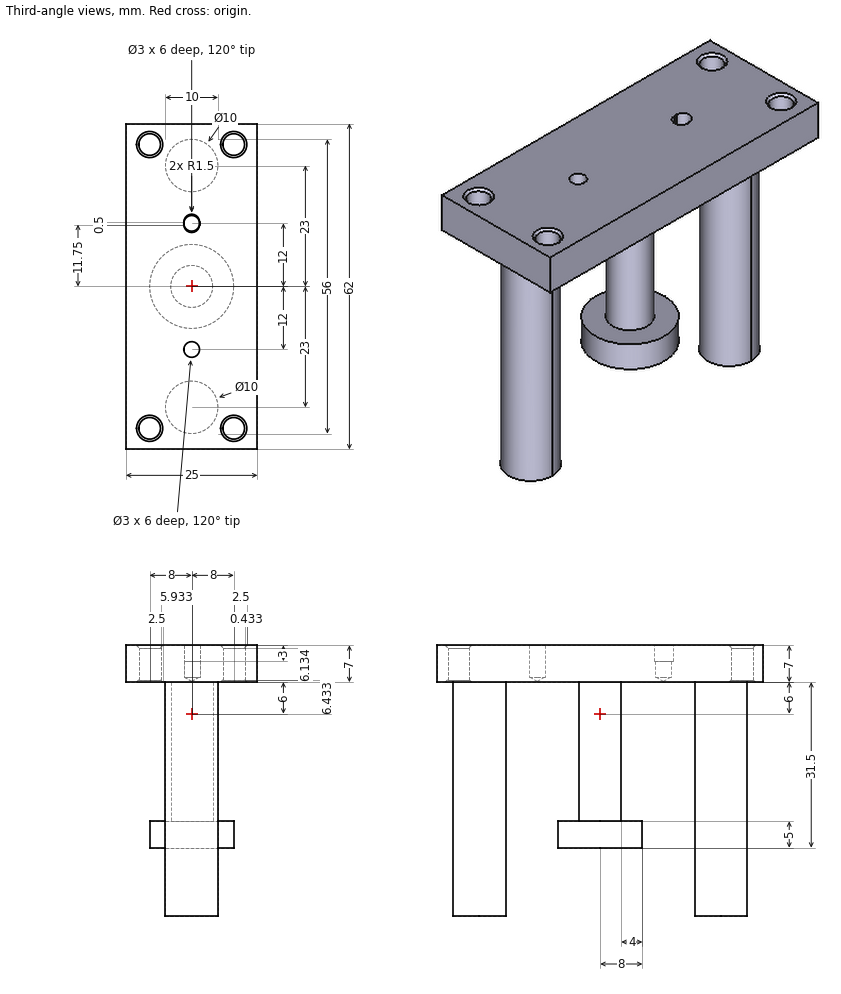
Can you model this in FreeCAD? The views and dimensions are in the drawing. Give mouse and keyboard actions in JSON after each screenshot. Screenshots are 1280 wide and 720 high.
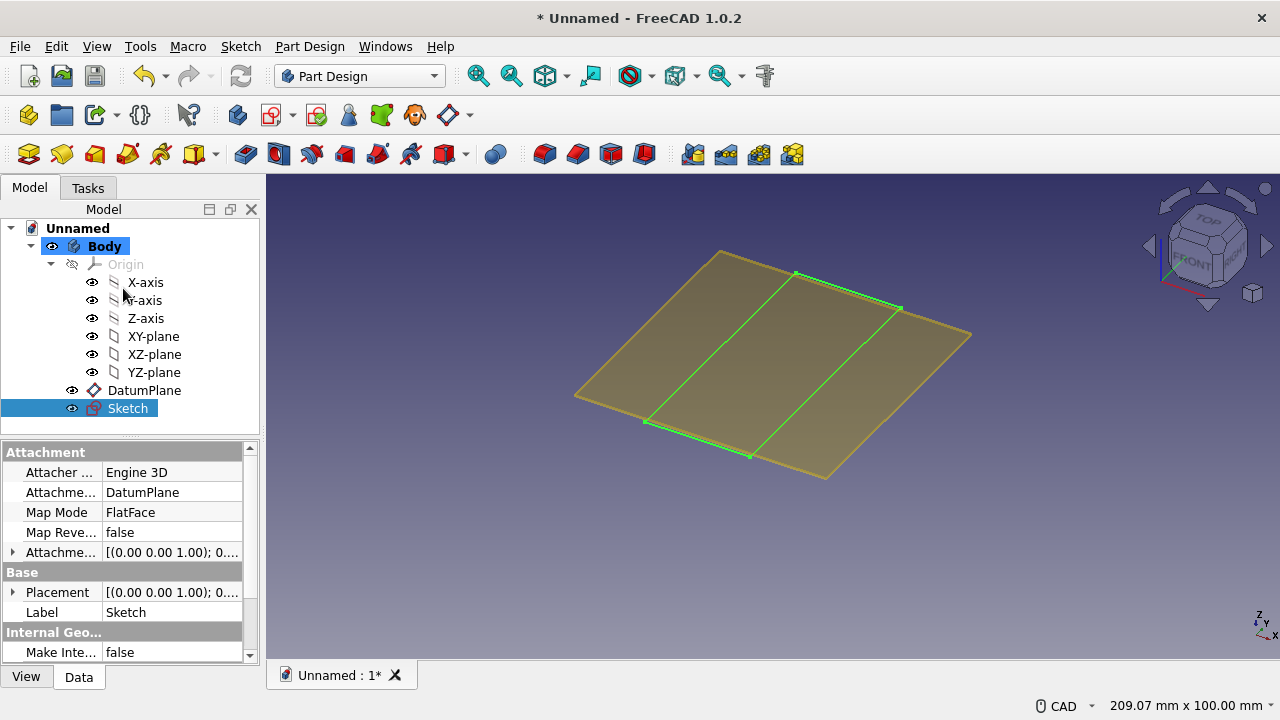
{"action": "left_click", "coordinate": [29, 154]}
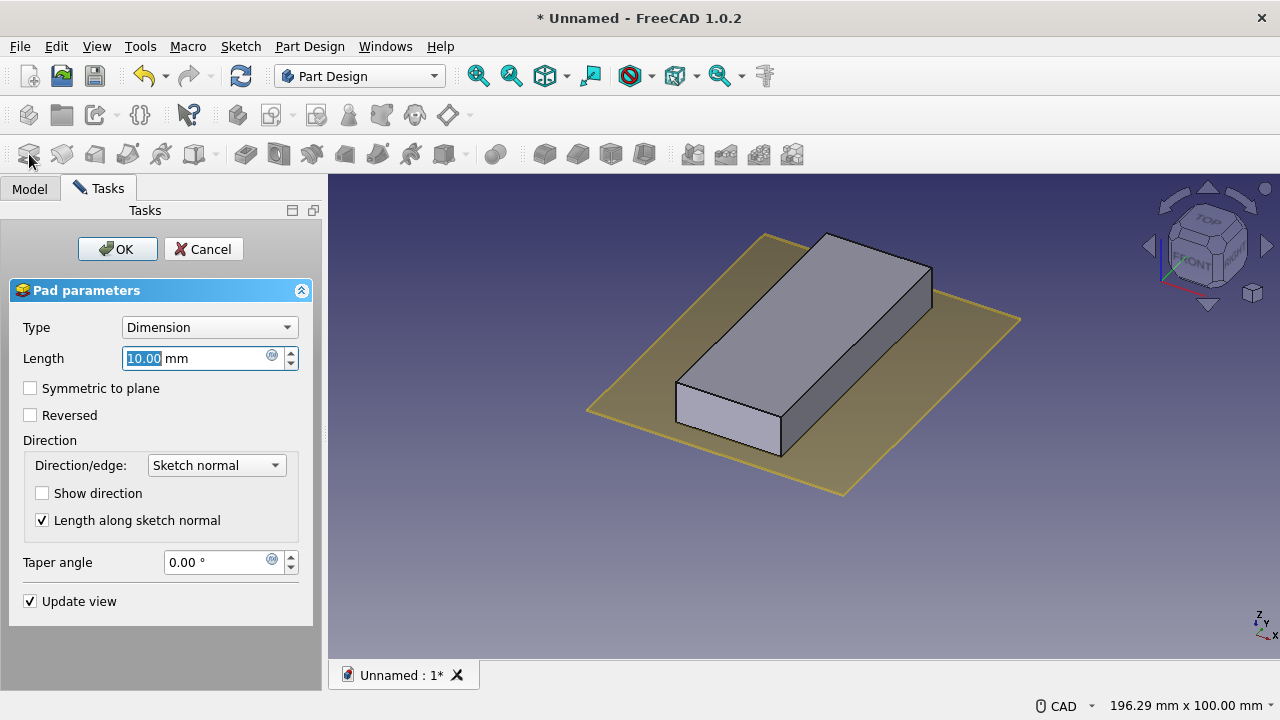
{"action": "type", "text": "7"}
{"action": "key", "text": "Tab"}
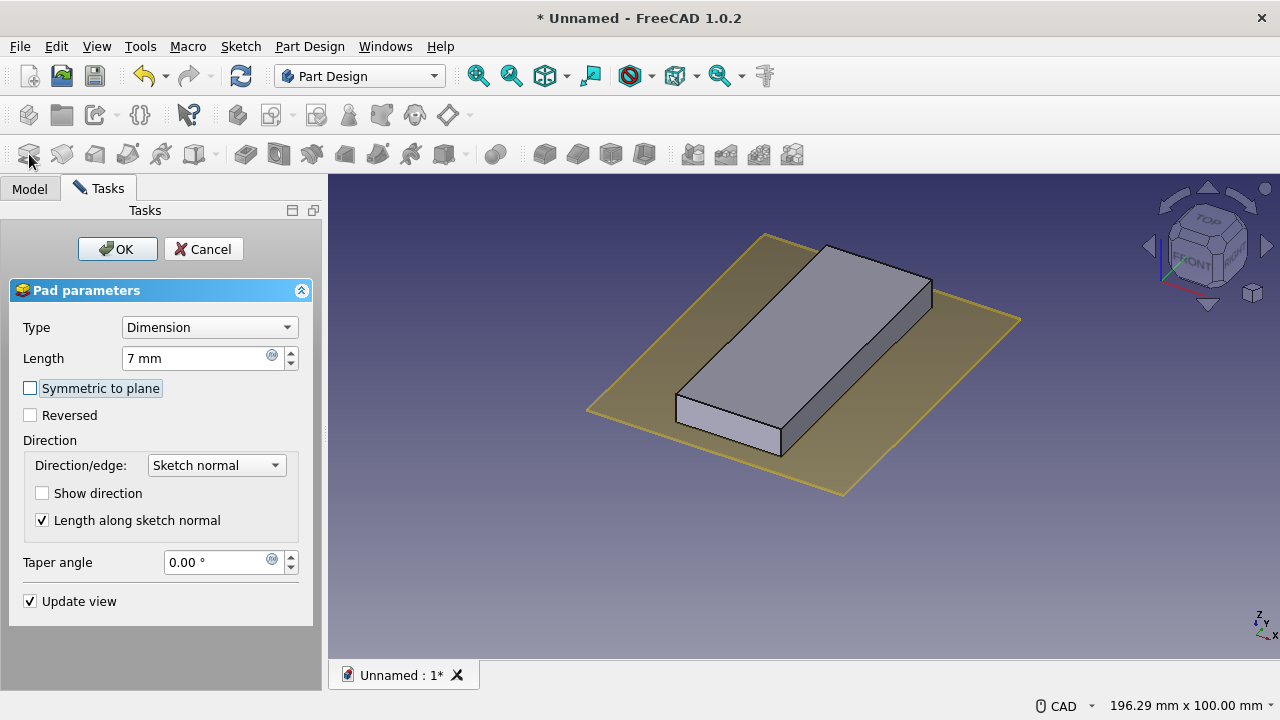
{"action": "left_click", "coordinate": [31, 415]}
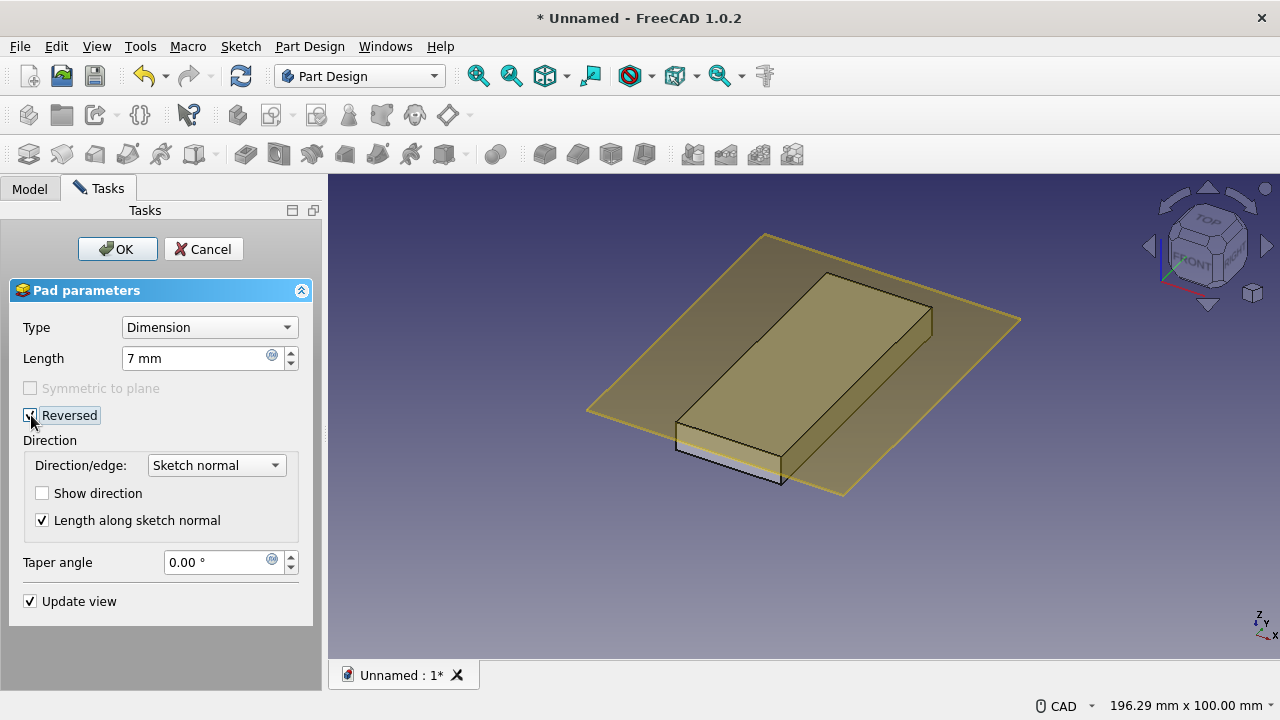
{"action": "left_click", "coordinate": [118, 249]}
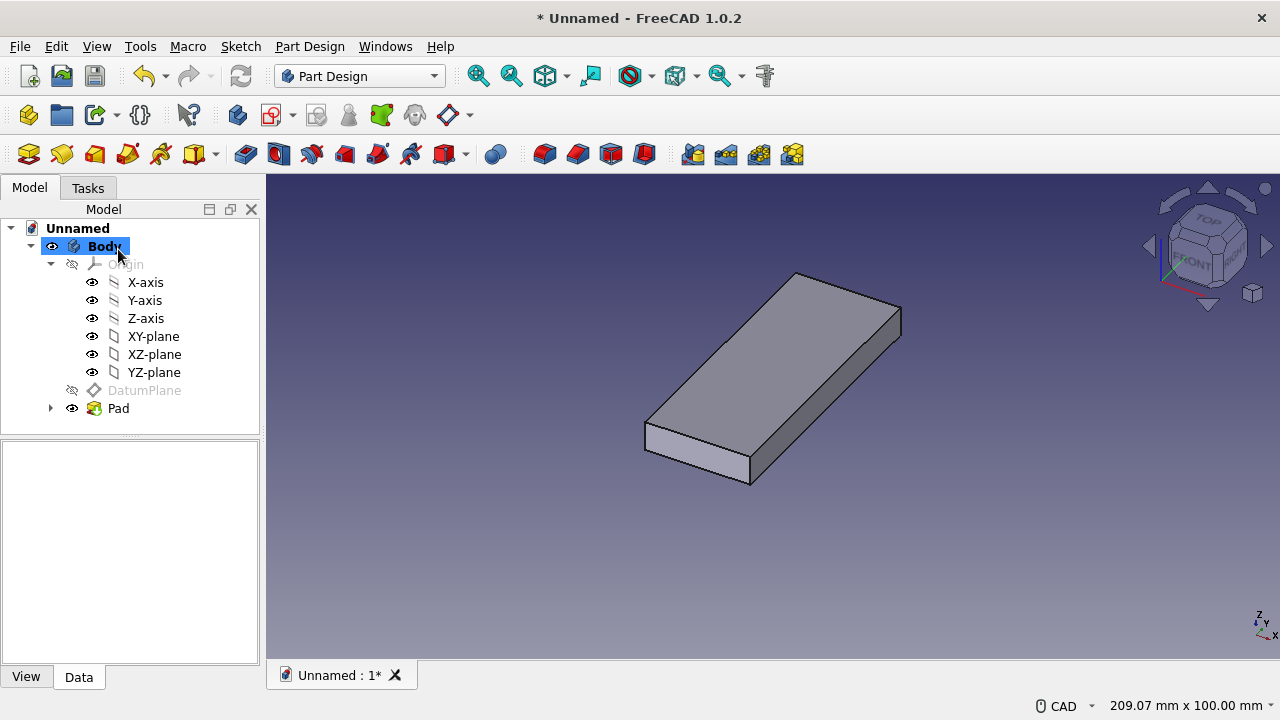
{"action": "left_click", "coordinate": [479, 76]}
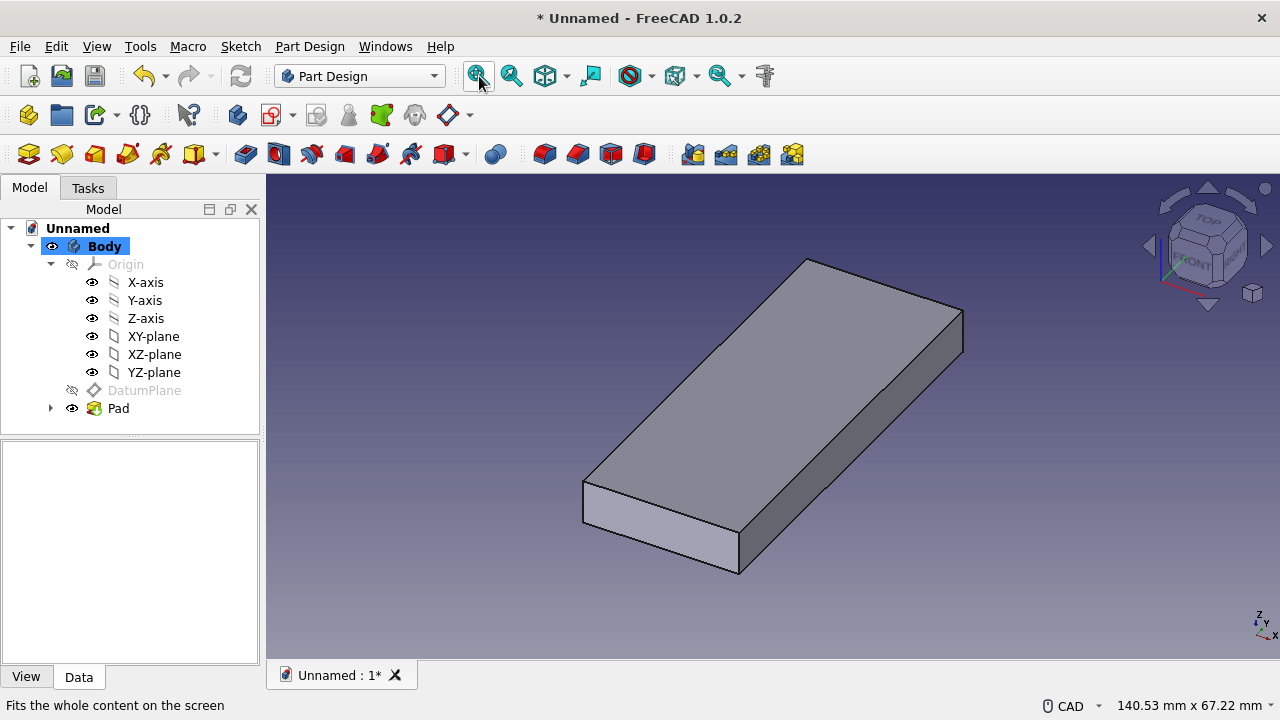
{"action": "left_click", "coordinate": [837, 331]}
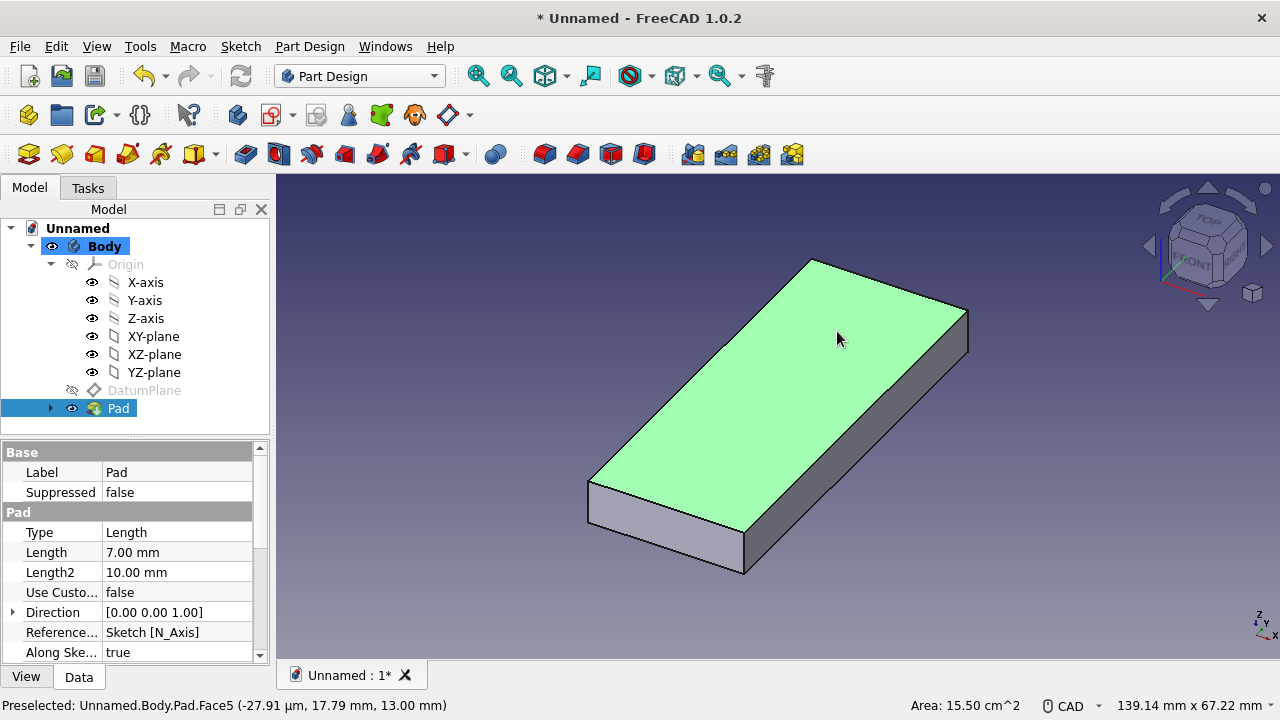
{"action": "left_click", "coordinate": [270, 116]}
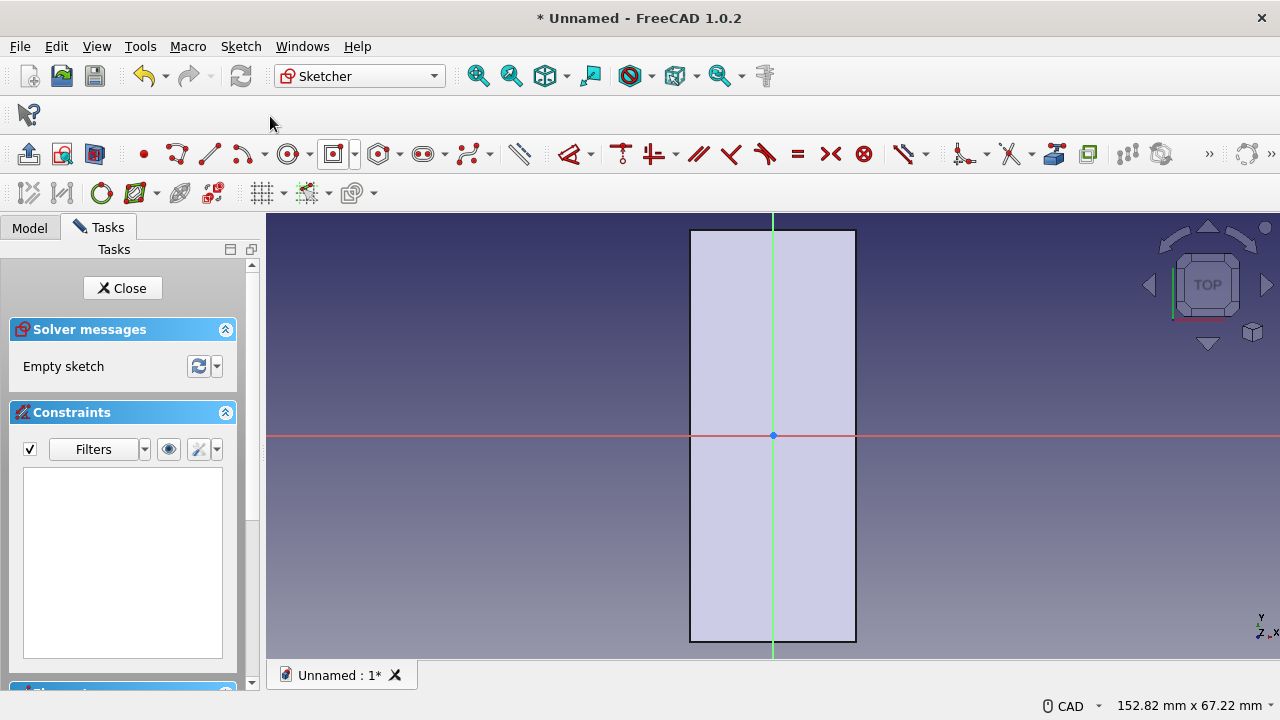
{"action": "scroll", "coordinate": [795, 241], "scroll_direction": "up", "scroll_amount": 7}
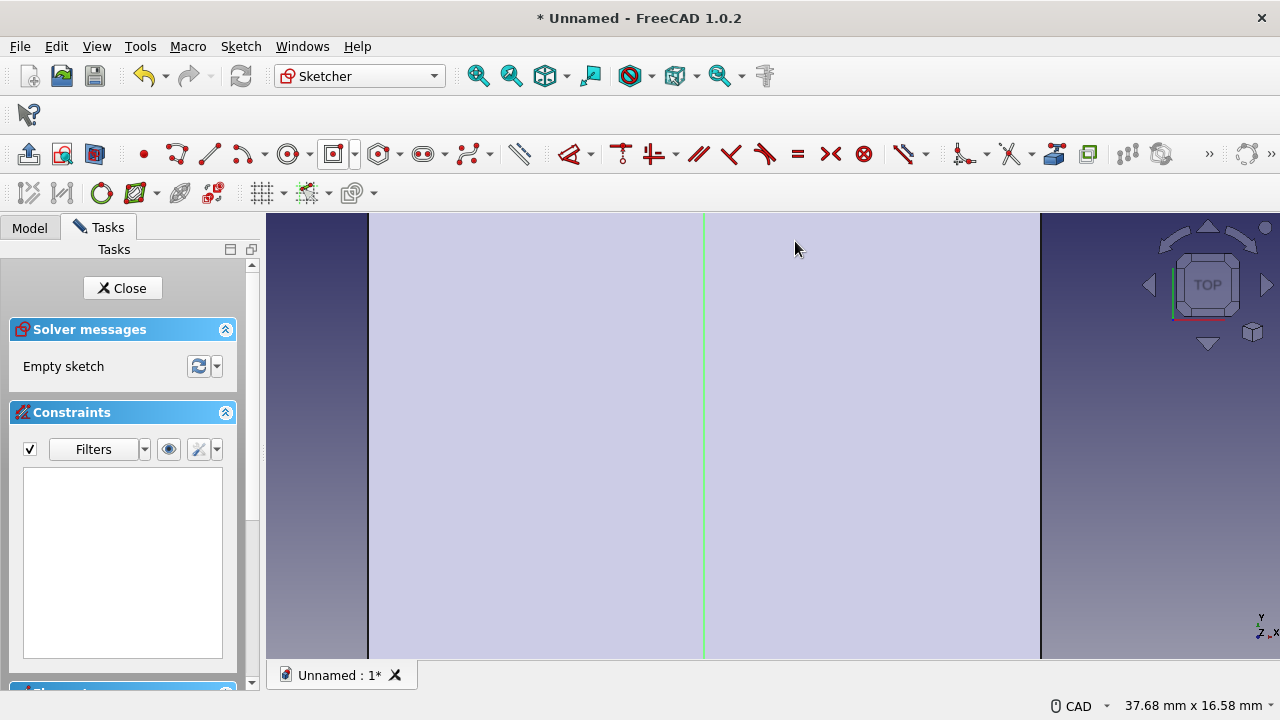
{"action": "left_click", "coordinate": [288, 154]}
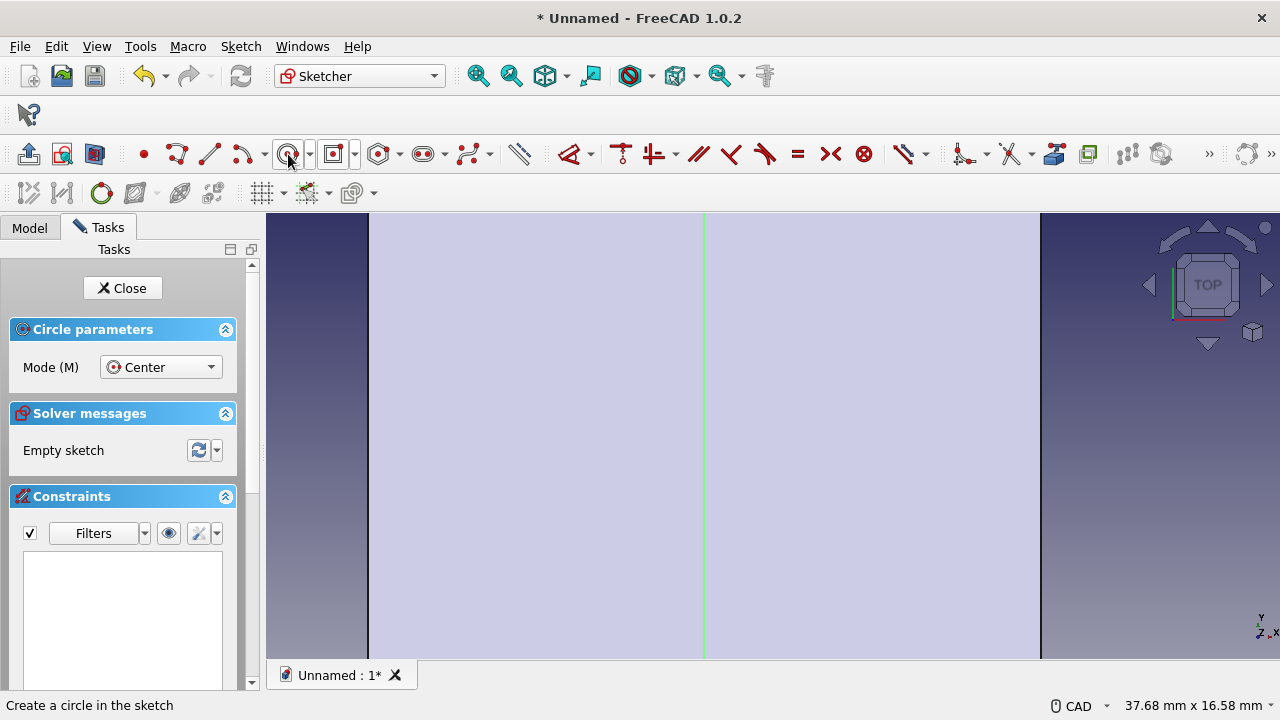
{"action": "left_click", "coordinate": [704, 413]}
{"action": "left_click", "coordinate": [799, 318]}
{"action": "key", "text": "Escape"}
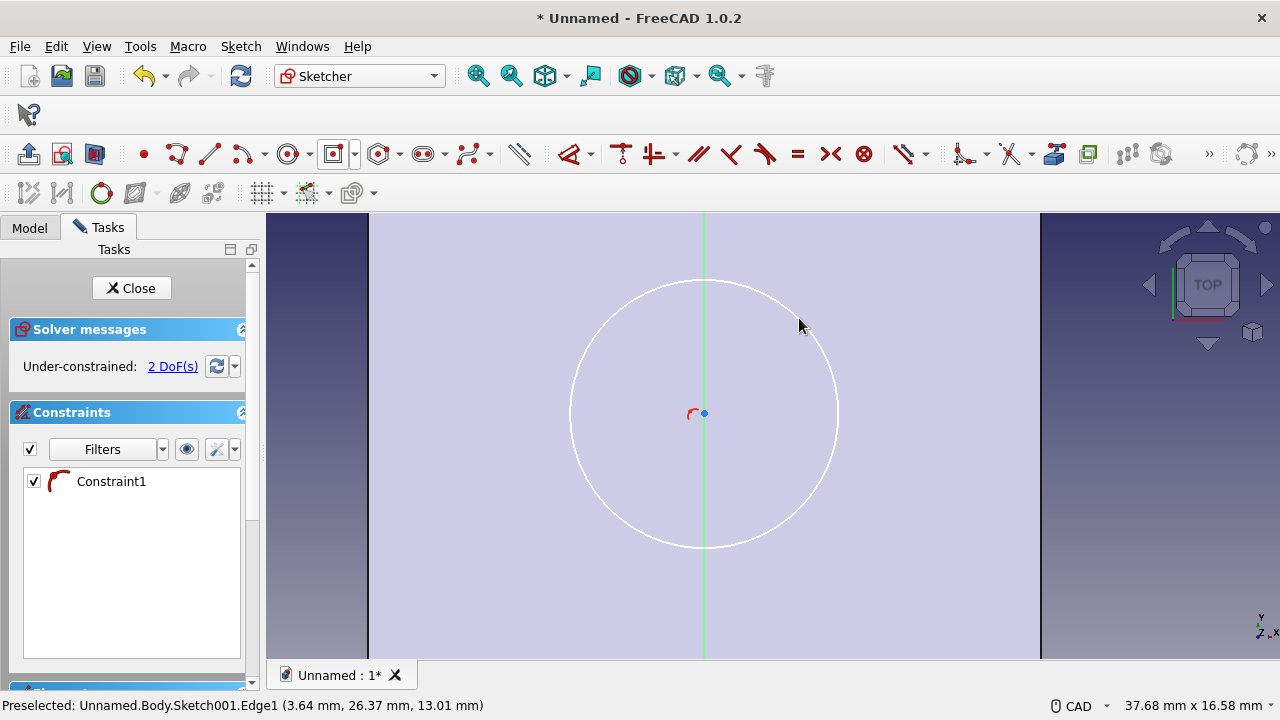
{"action": "left_click", "coordinate": [568, 154]}